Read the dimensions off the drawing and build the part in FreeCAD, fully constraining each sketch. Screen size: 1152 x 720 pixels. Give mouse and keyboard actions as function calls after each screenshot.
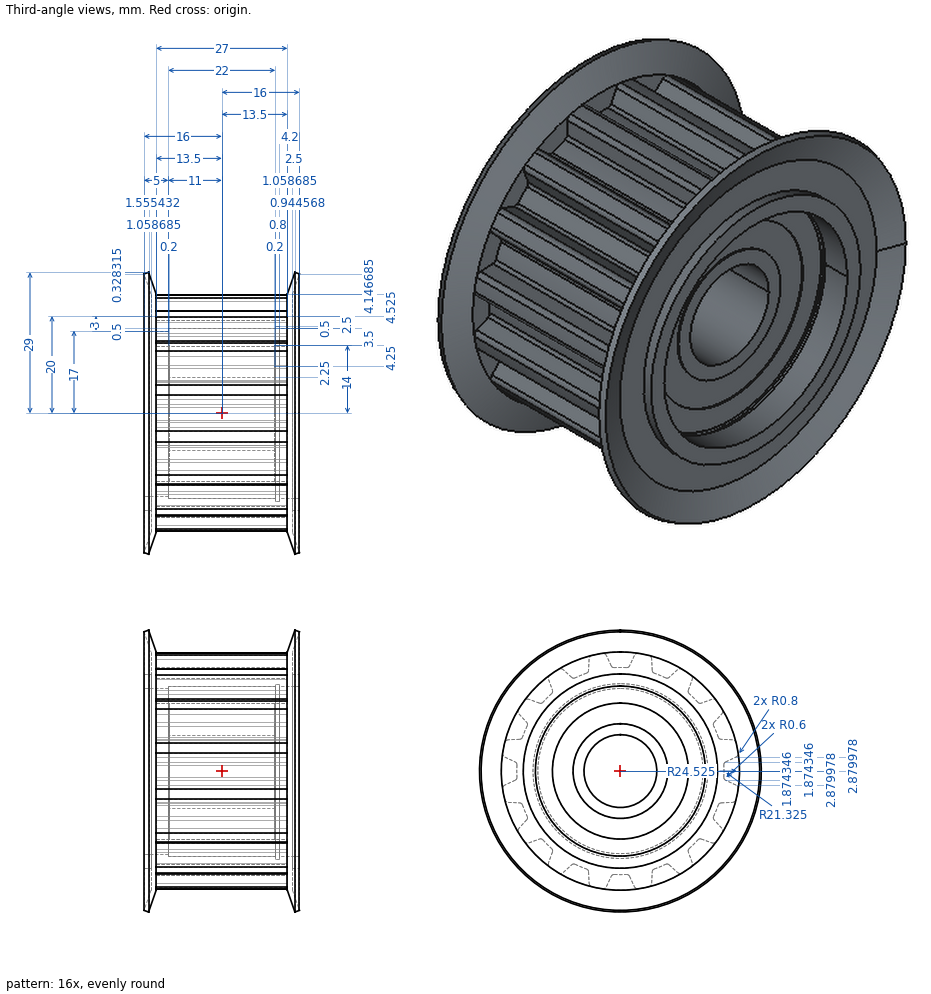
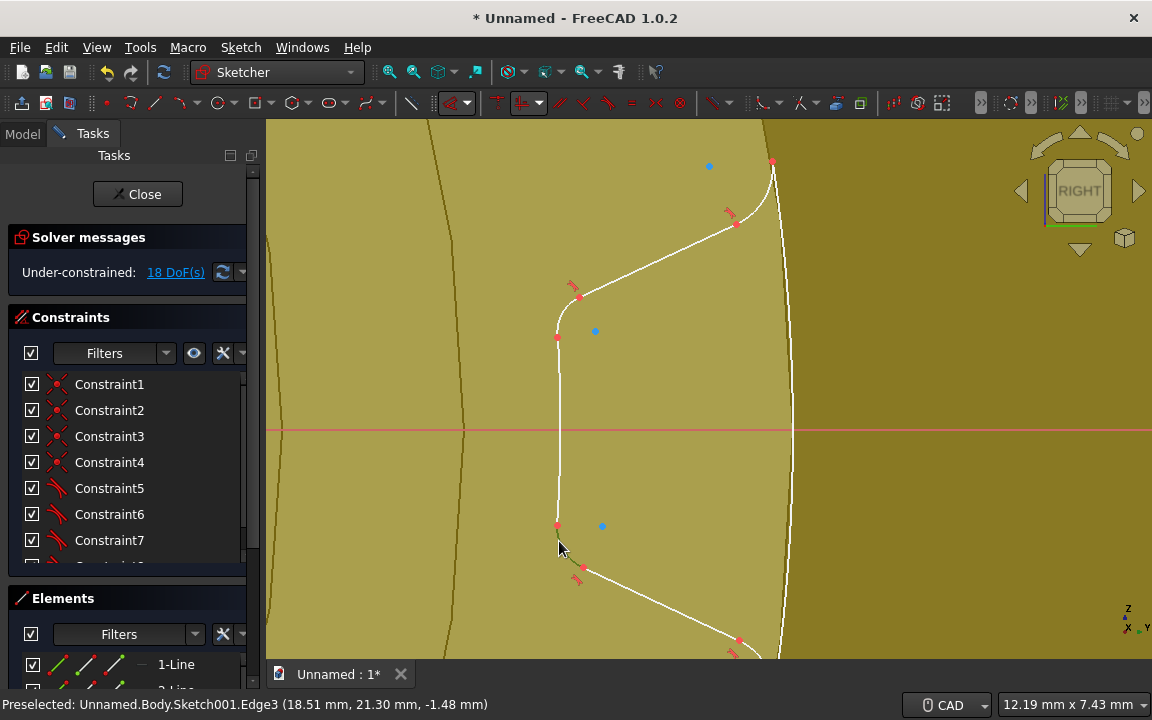
click(560, 469)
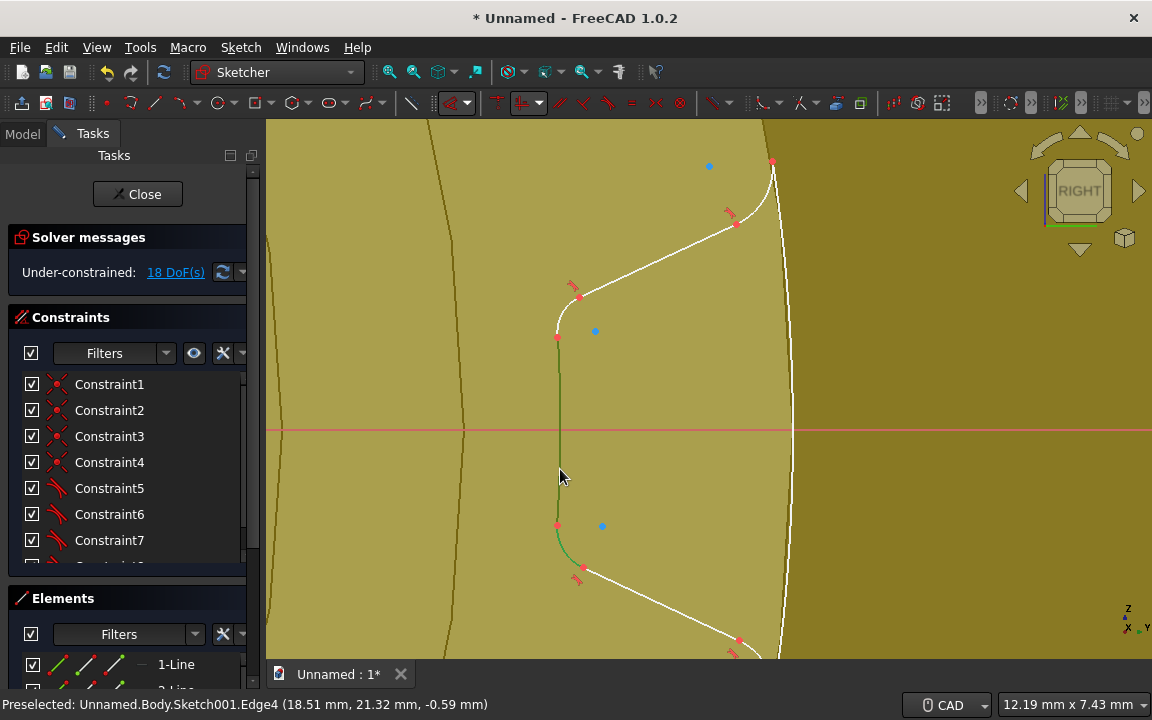
click(608, 104)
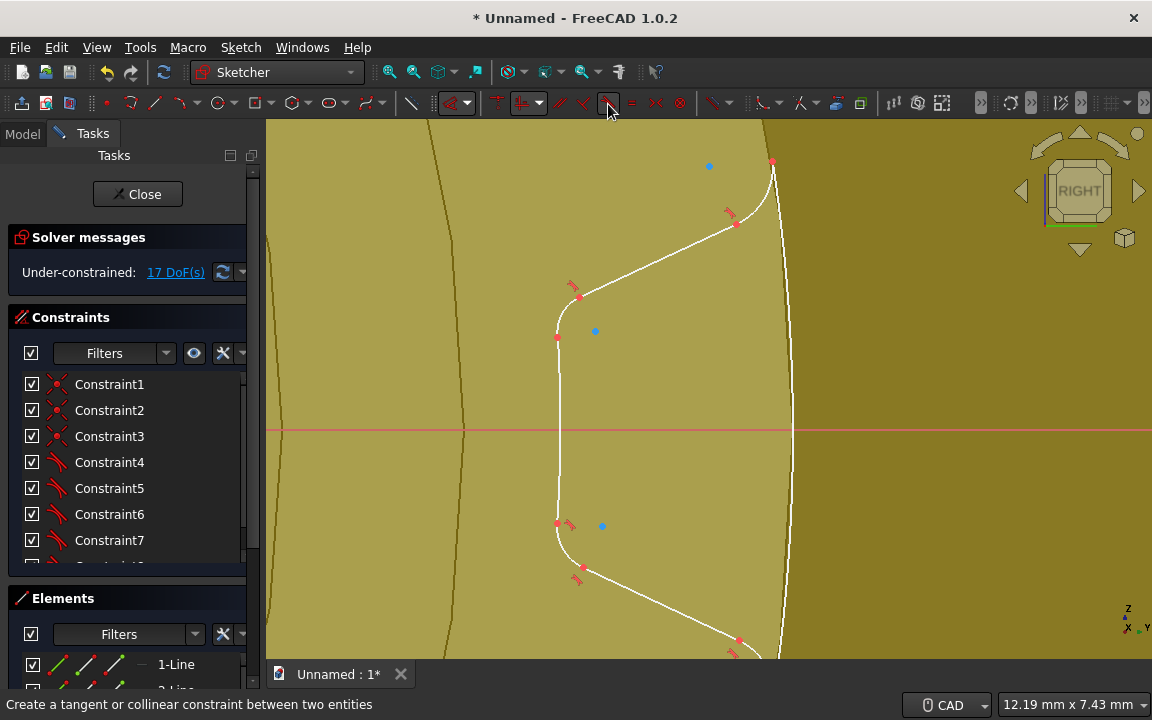
click(560, 468)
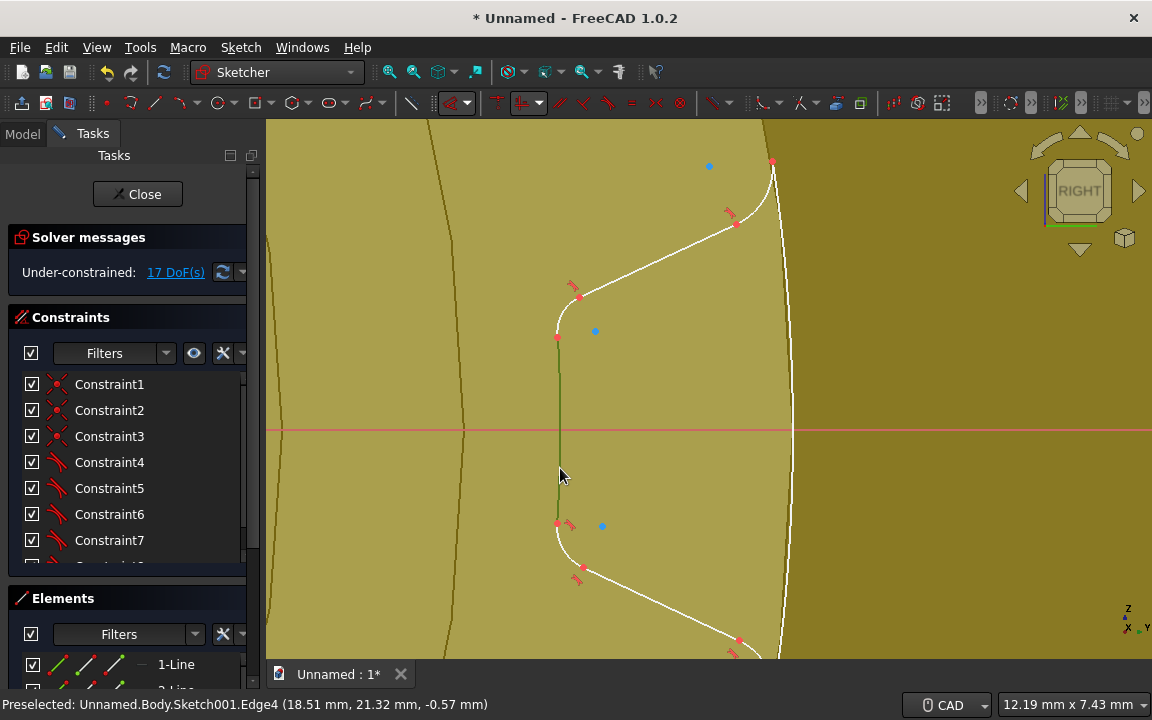
click(568, 306)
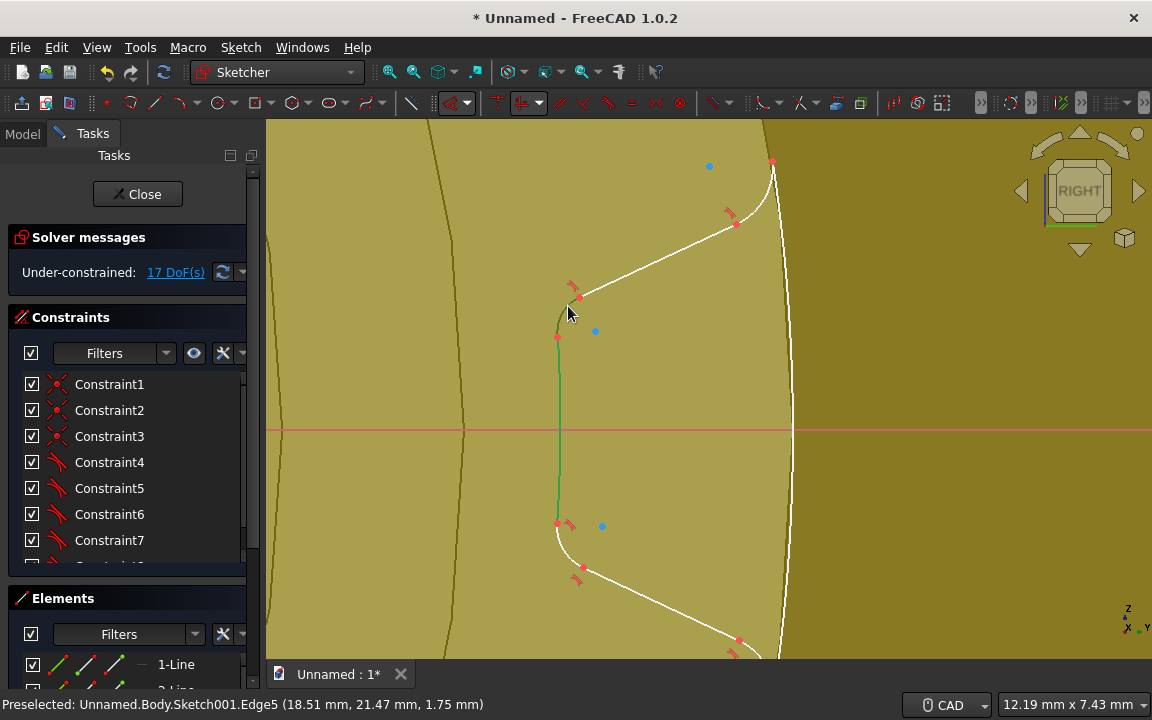
click(608, 104)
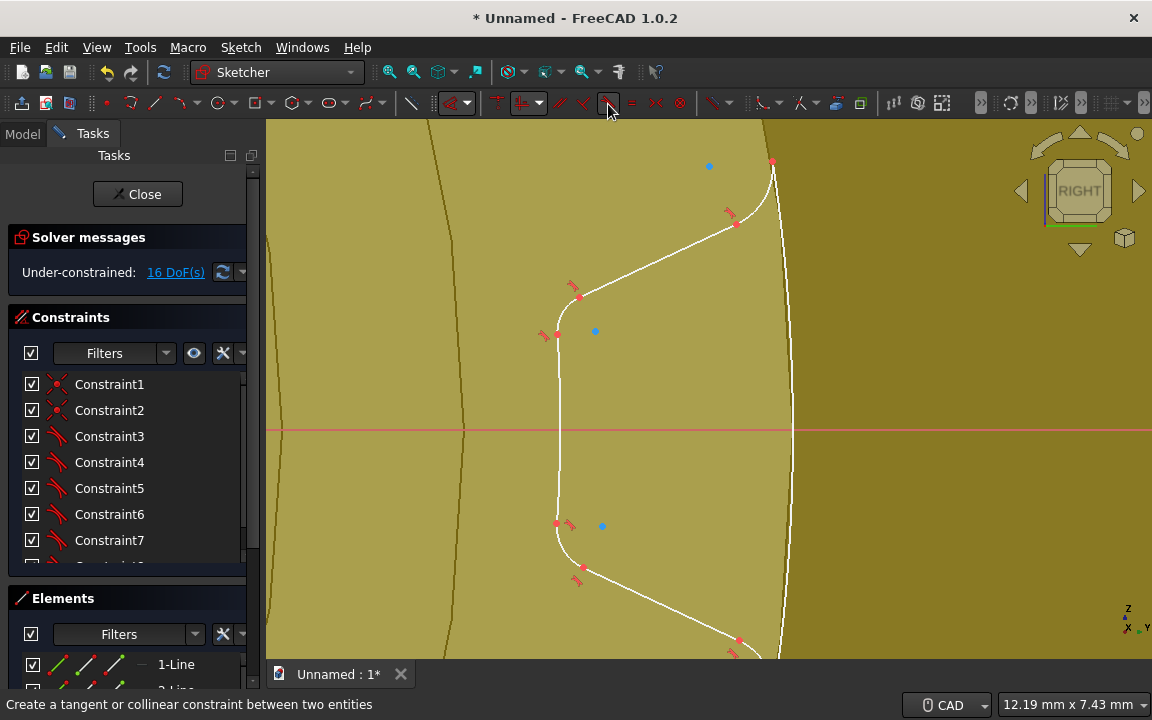
click(755, 211)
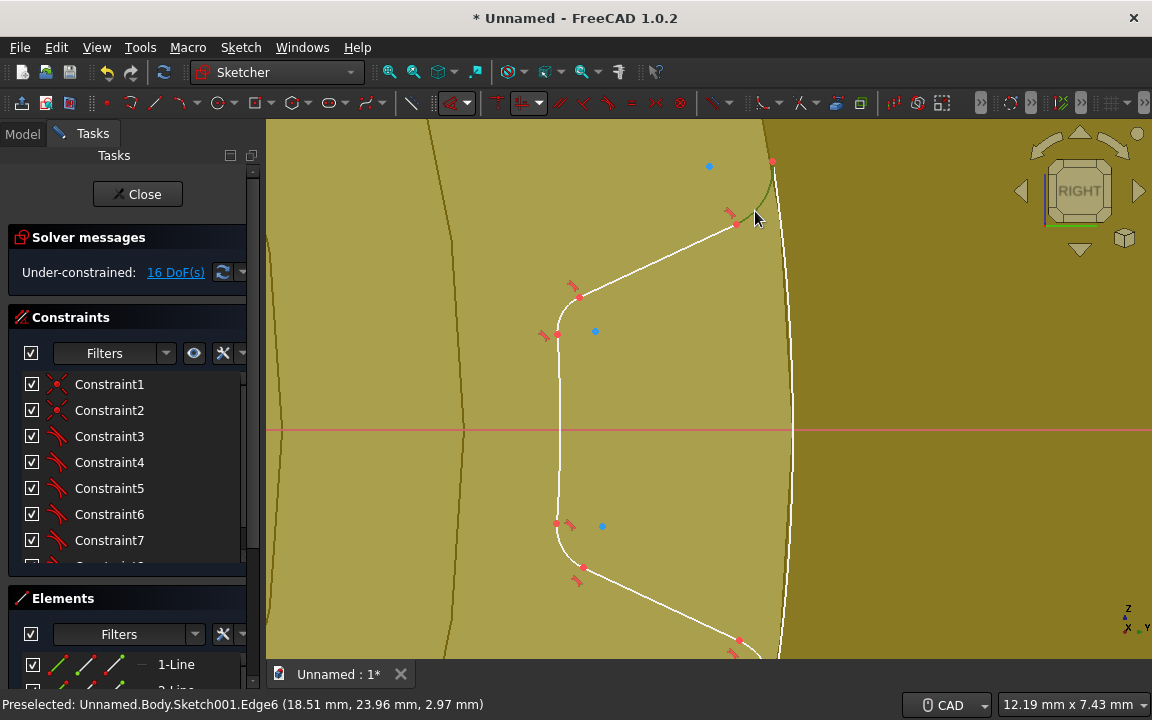
click(790, 541)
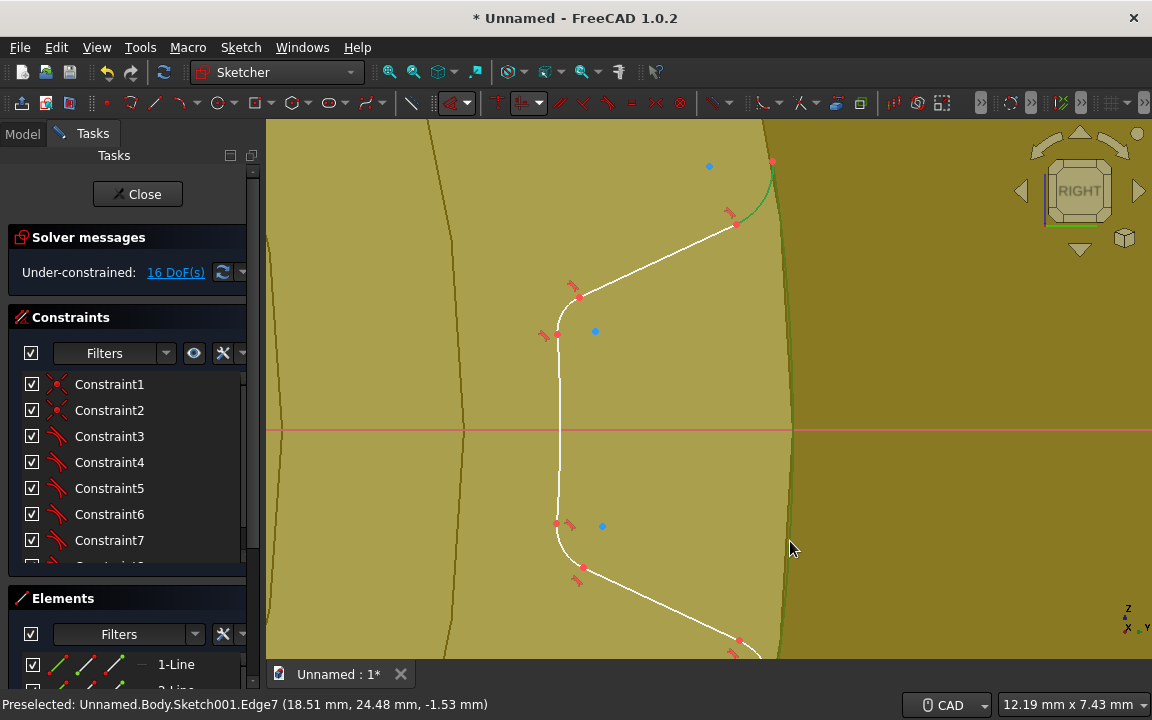
click(608, 104)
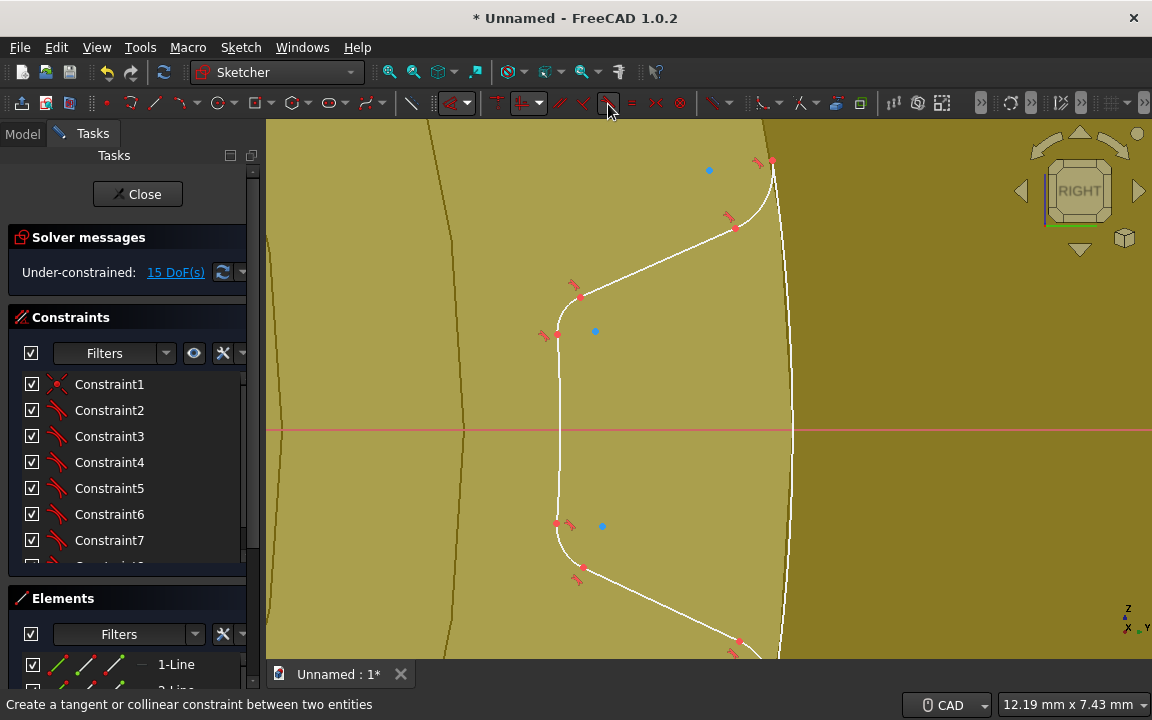
click(789, 541)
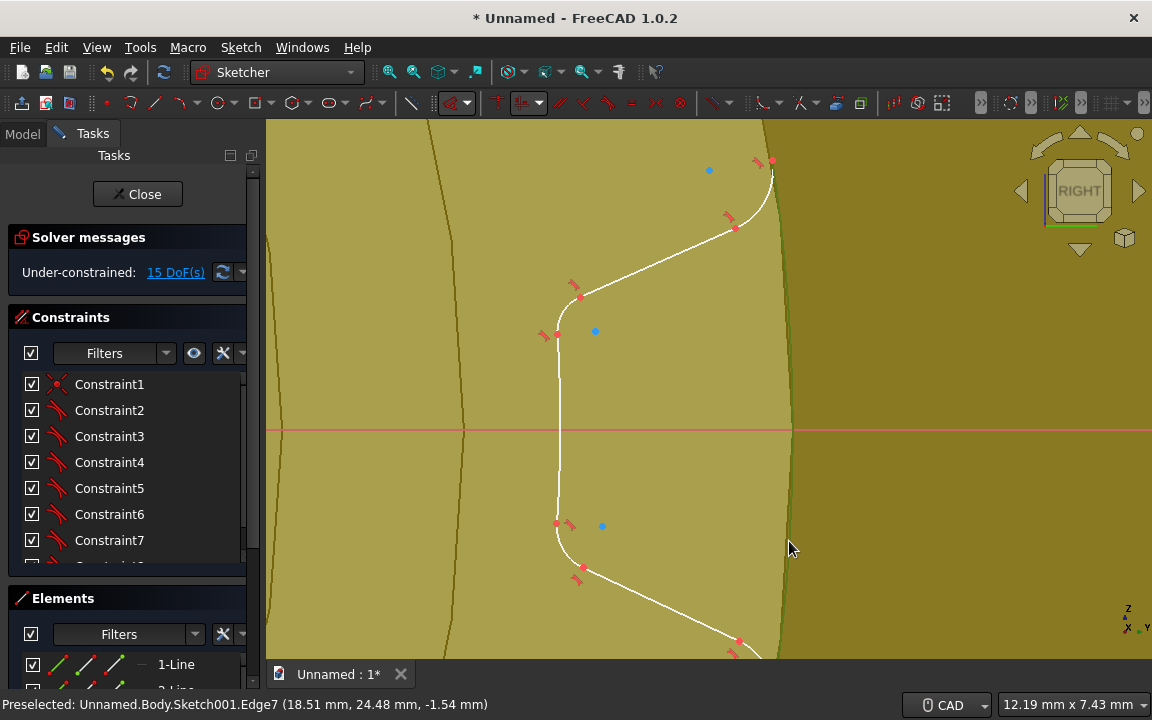
scroll(570, 305, down, 2)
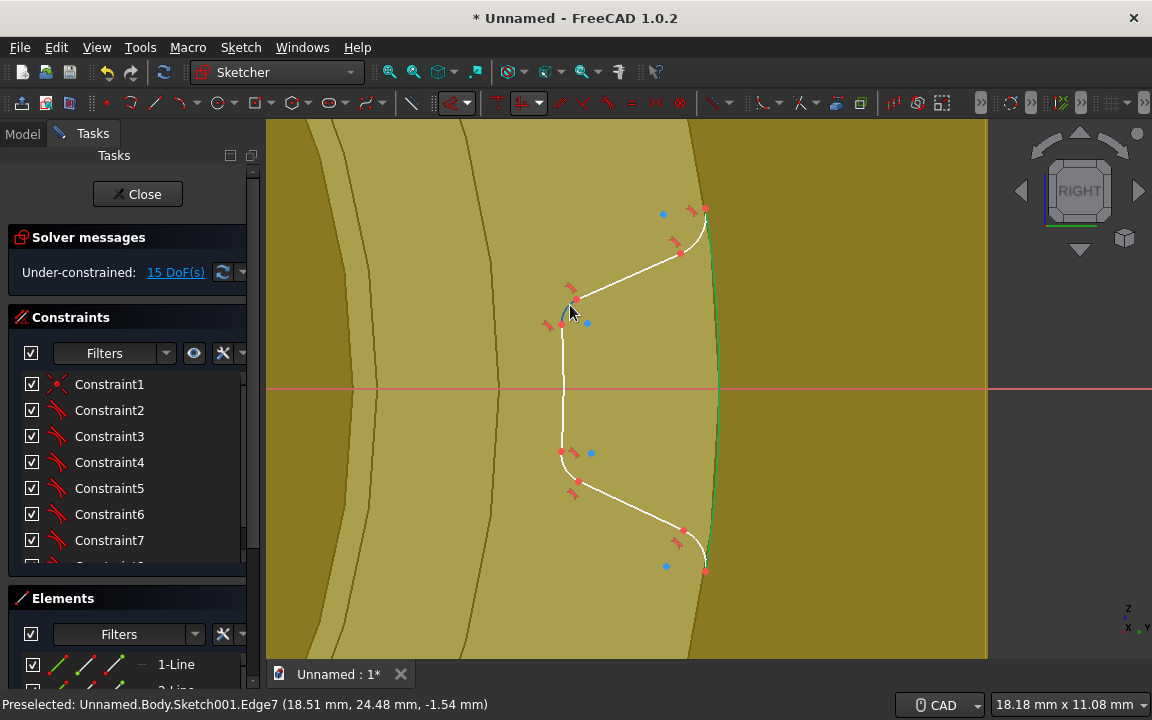
click(696, 539)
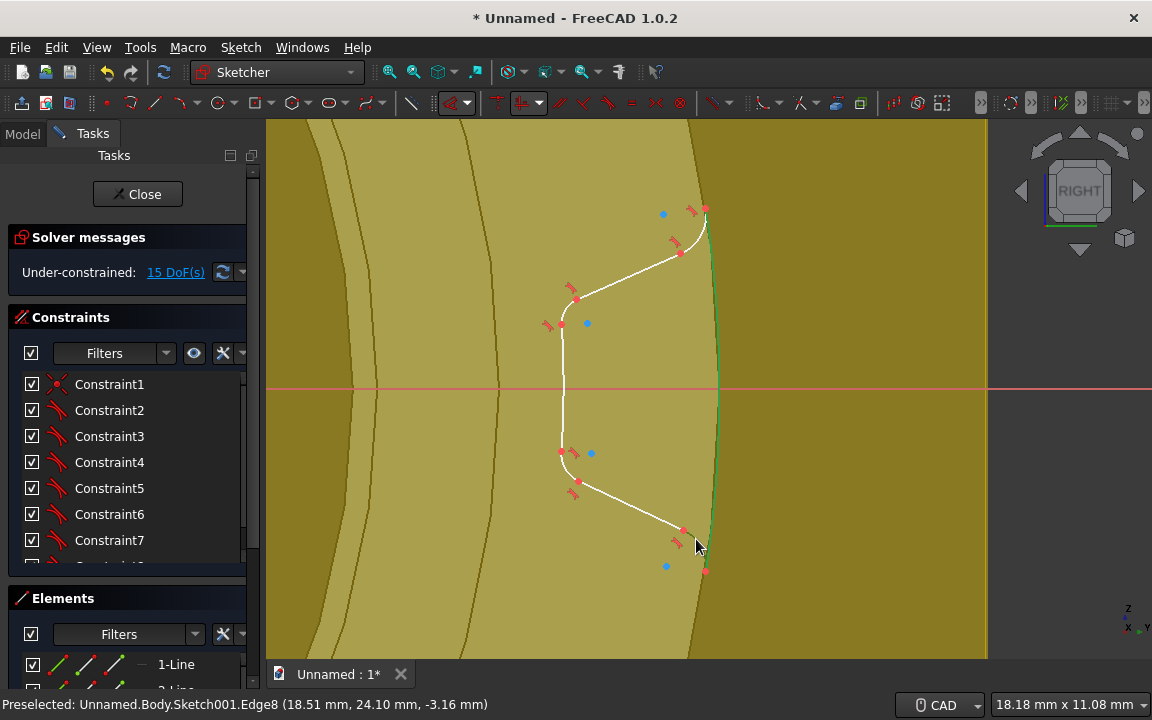
click(608, 104)